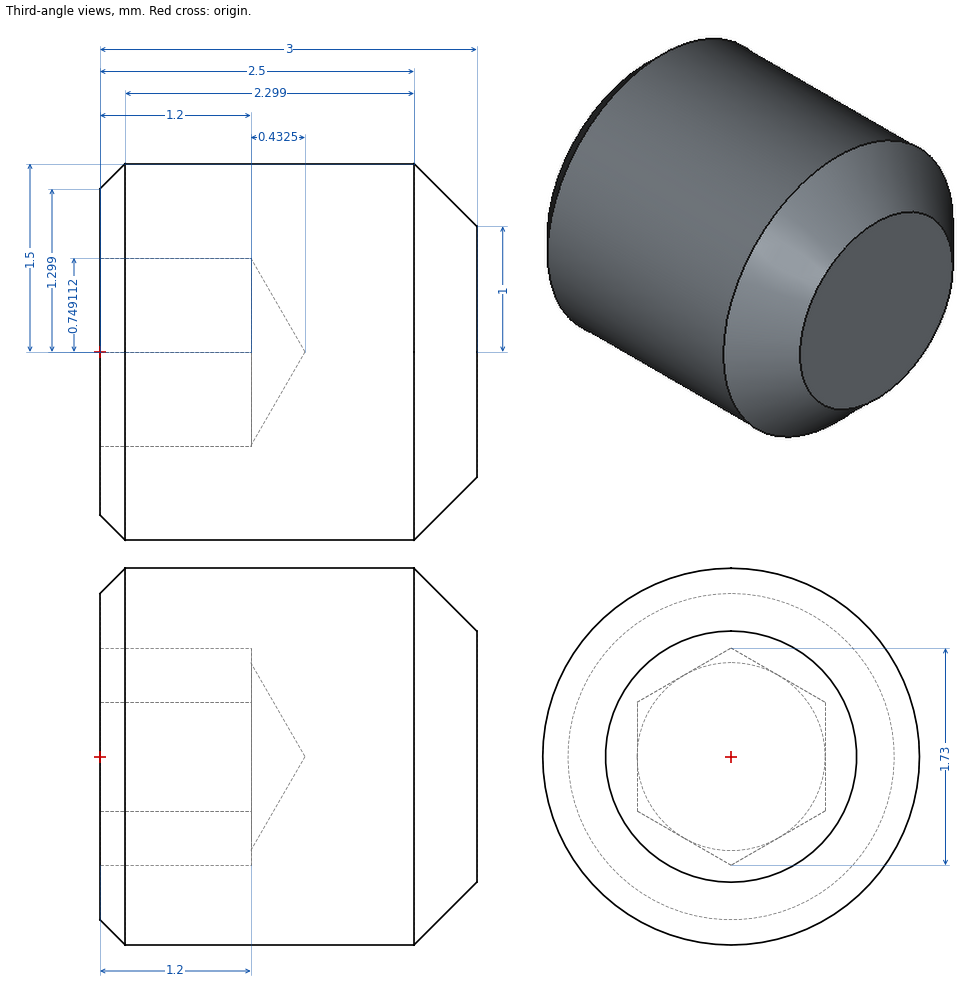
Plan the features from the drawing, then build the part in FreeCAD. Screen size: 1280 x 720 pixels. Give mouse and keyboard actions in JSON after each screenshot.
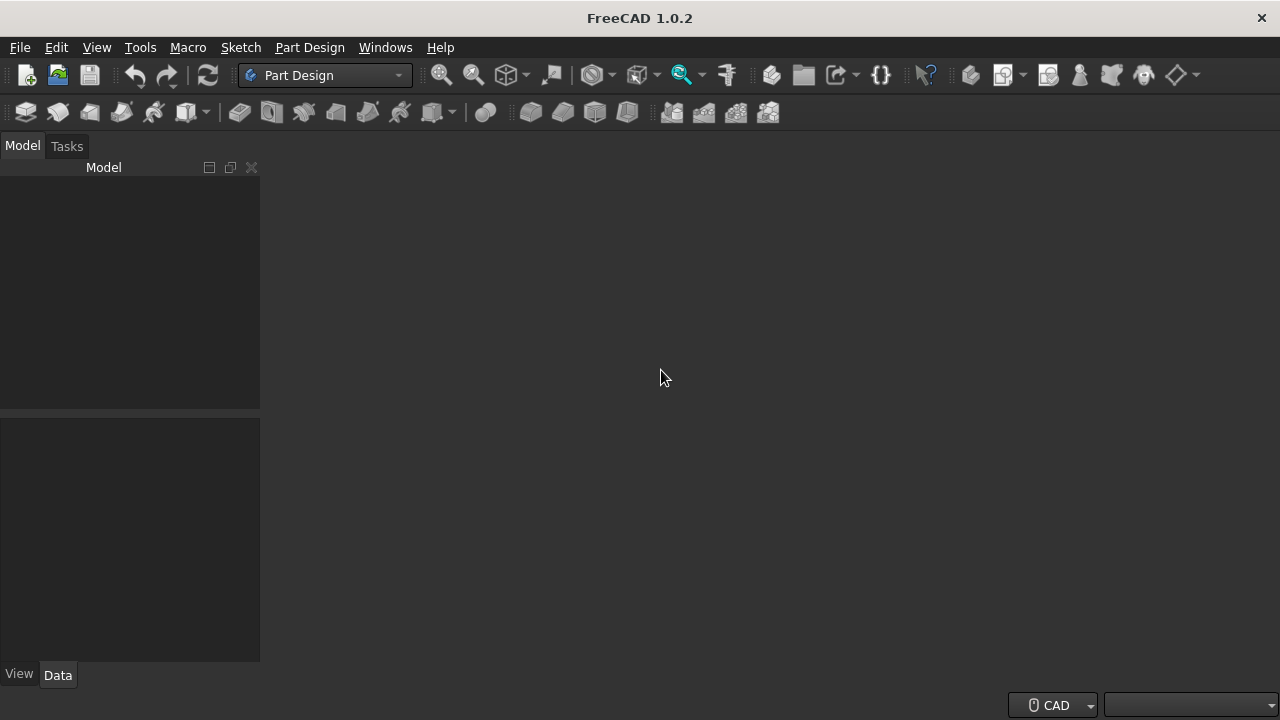
{"action": "left_click", "coordinate": [26, 76]}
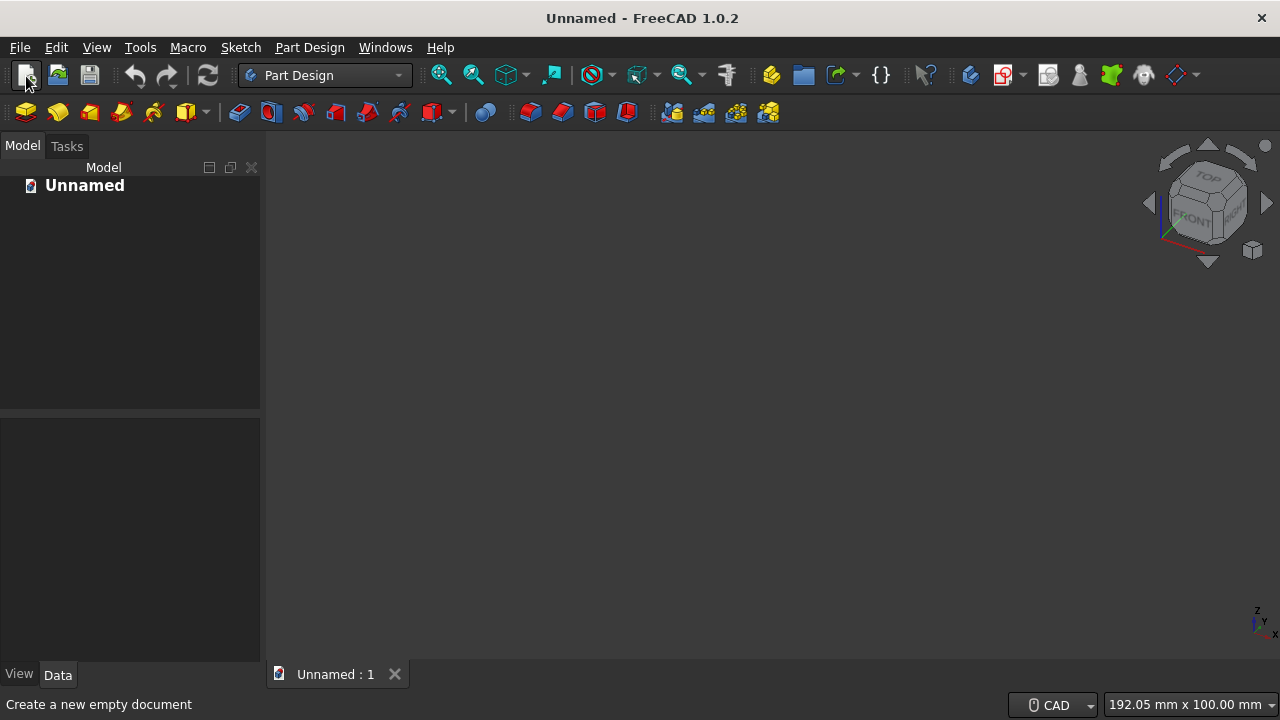
{"action": "left_click", "coordinate": [1004, 76]}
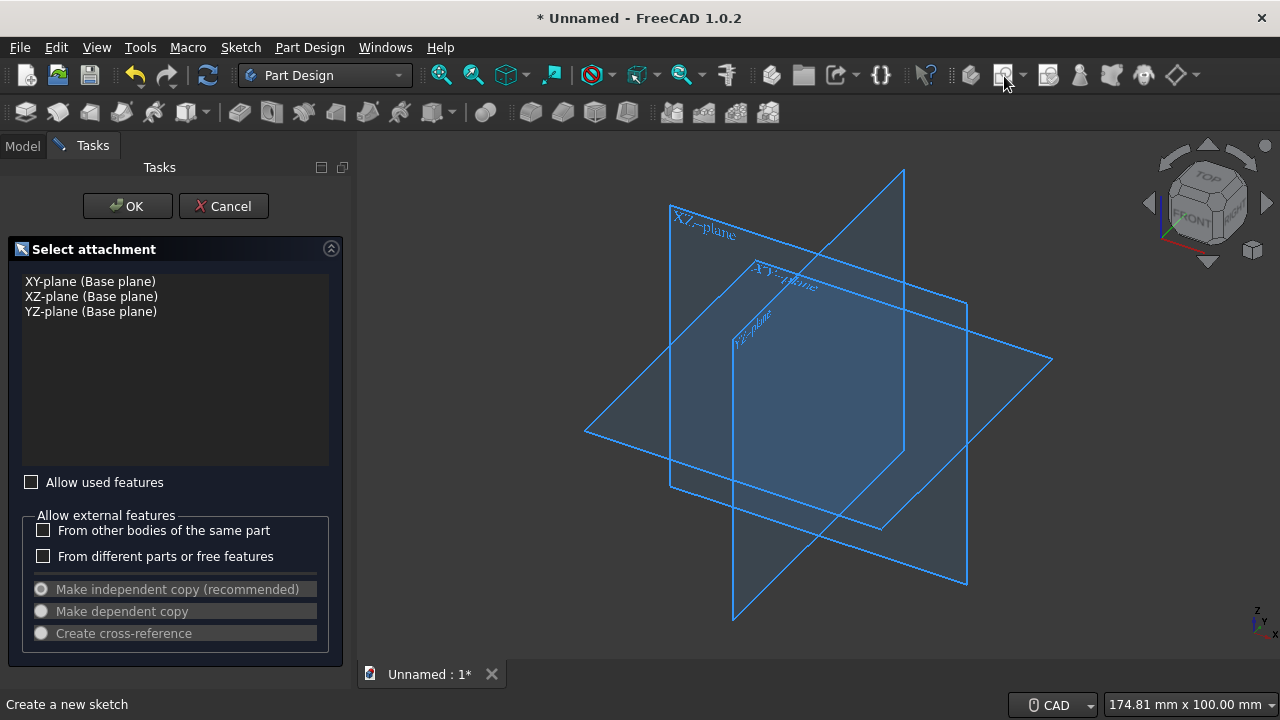
{"action": "left_click", "coordinate": [82, 282]}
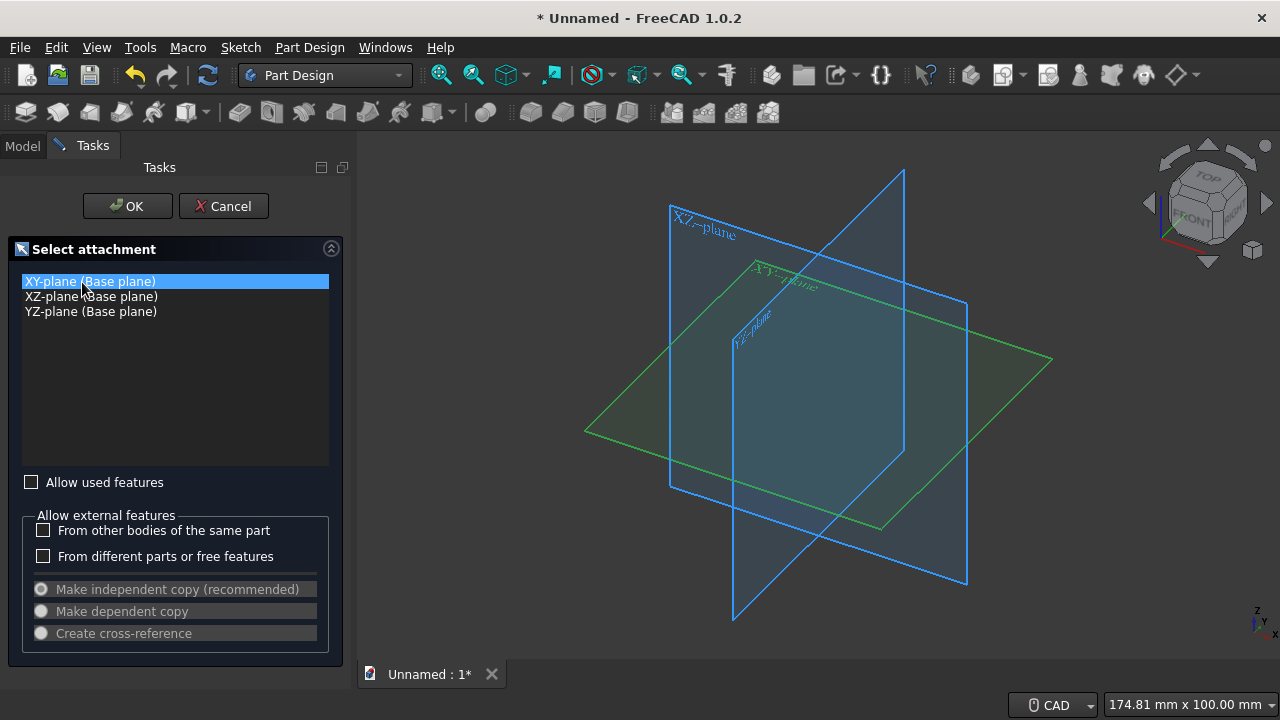
{"action": "left_click", "coordinate": [128, 206]}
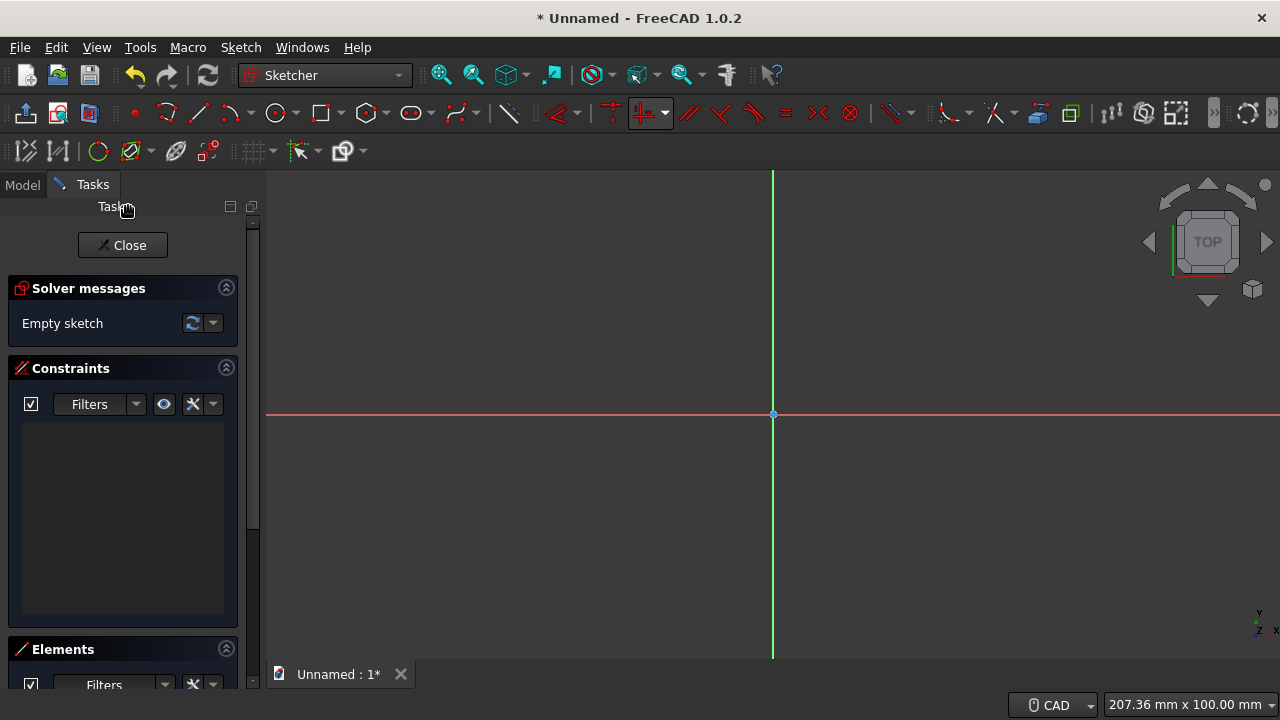
{"action": "scroll", "coordinate": [784, 411], "scroll_direction": "up", "scroll_amount": 15}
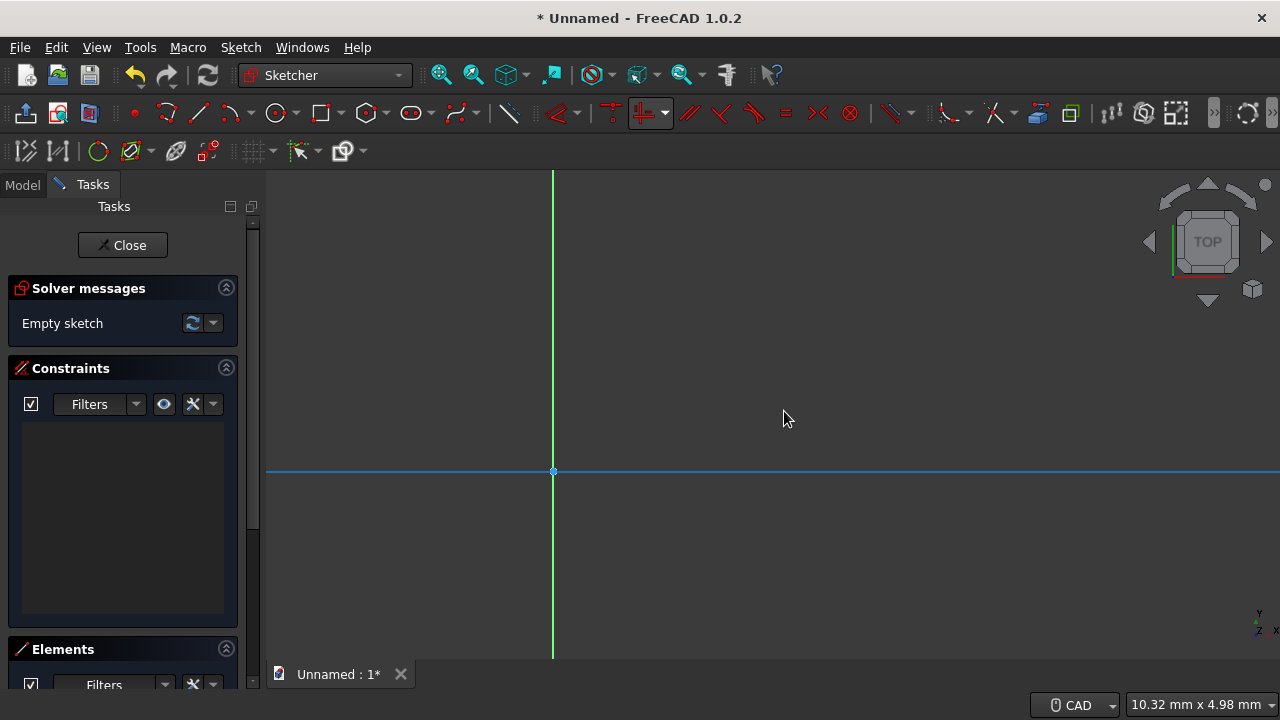
{"action": "scroll", "coordinate": [696, 378], "scroll_direction": "up", "scroll_amount": 3}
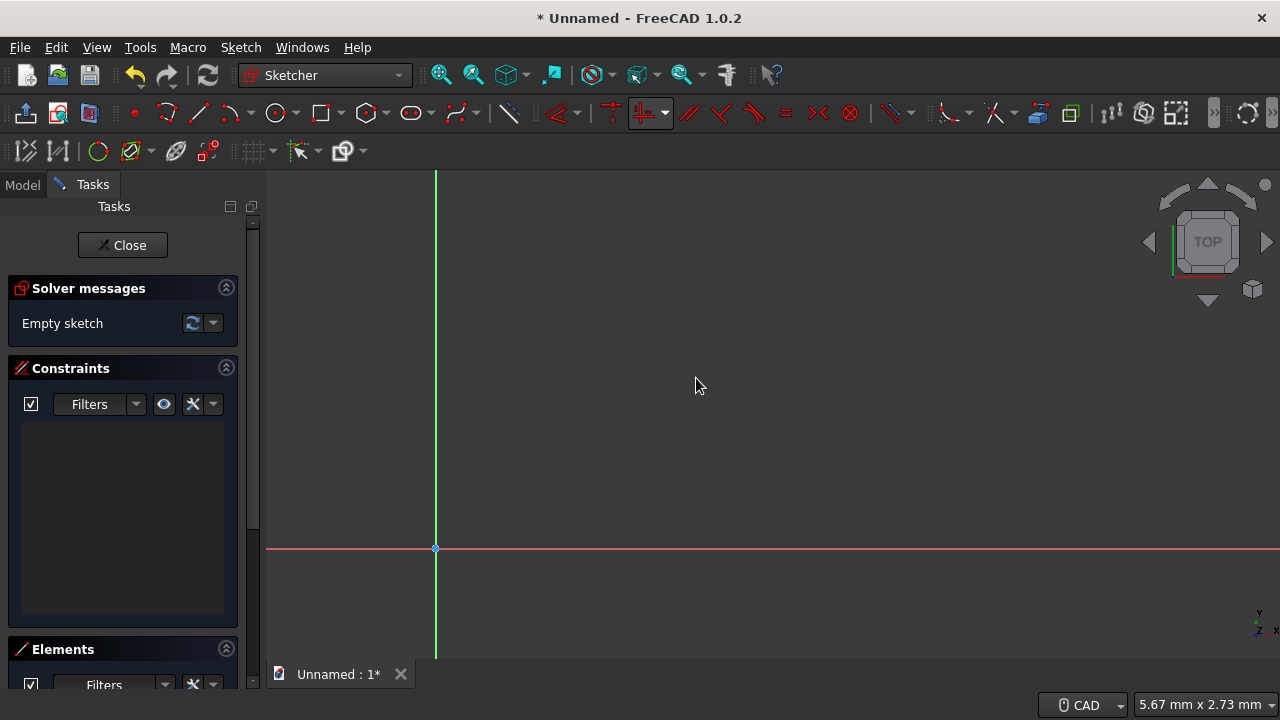
{"action": "left_click", "coordinate": [168, 114]}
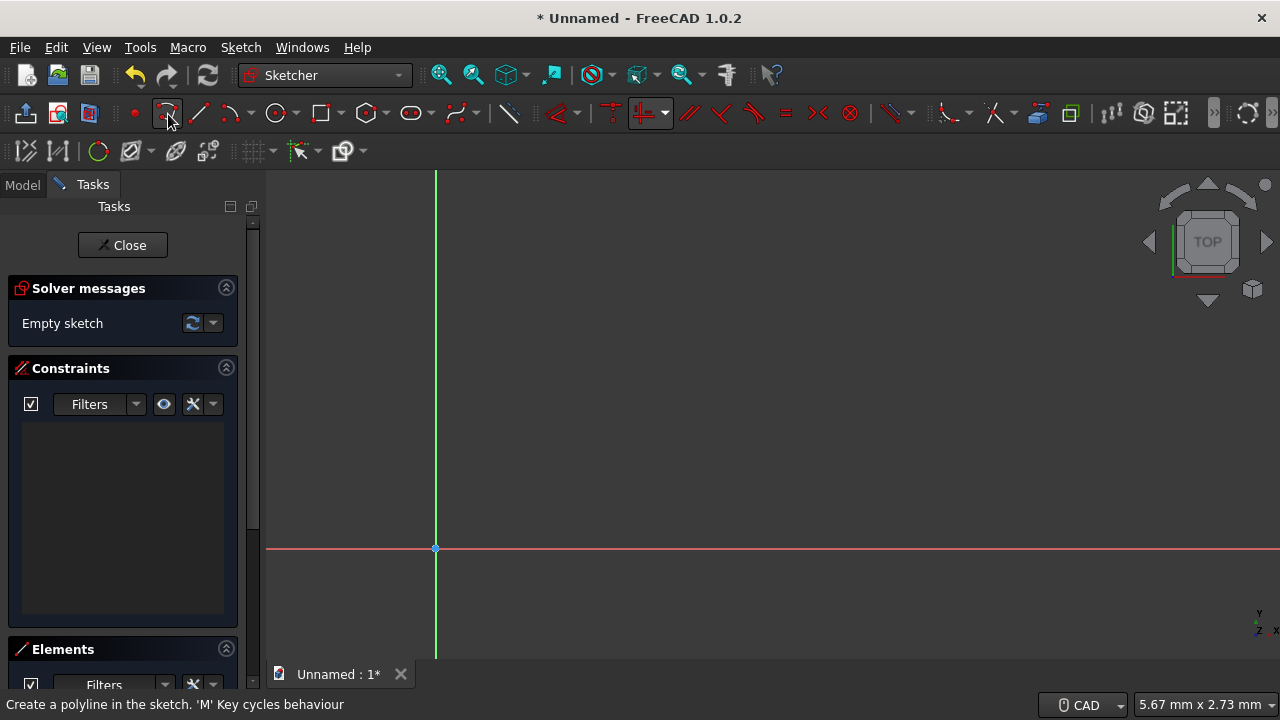
{"action": "left_click", "coordinate": [436, 549]}
{"action": "left_click", "coordinate": [973, 540]}
{"action": "left_click", "coordinate": [973, 370]}
{"action": "left_click", "coordinate": [883, 280]}
{"action": "left_click", "coordinate": [472, 280]}
{"action": "left_click", "coordinate": [445, 316]}
{"action": "left_click", "coordinate": [436, 549]}
{"action": "key", "text": "Escape"}
{"action": "key", "text": "Escape"}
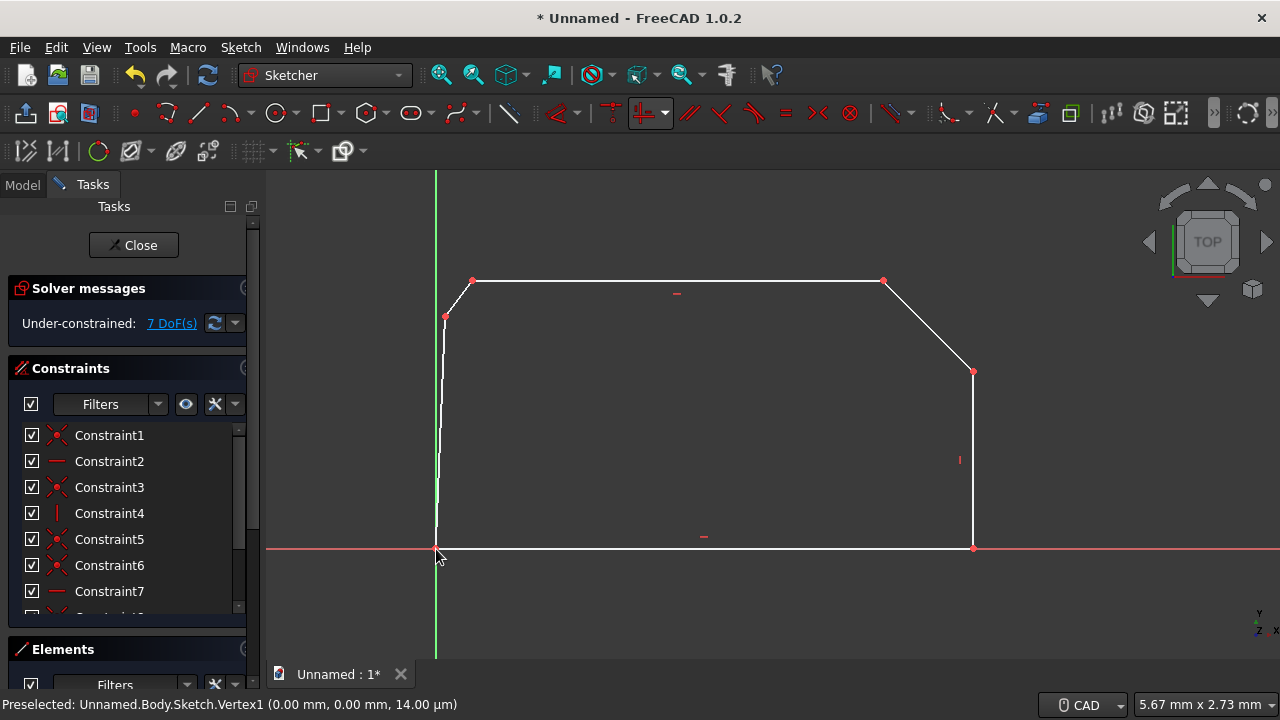
{"action": "left_click", "coordinate": [438, 479]}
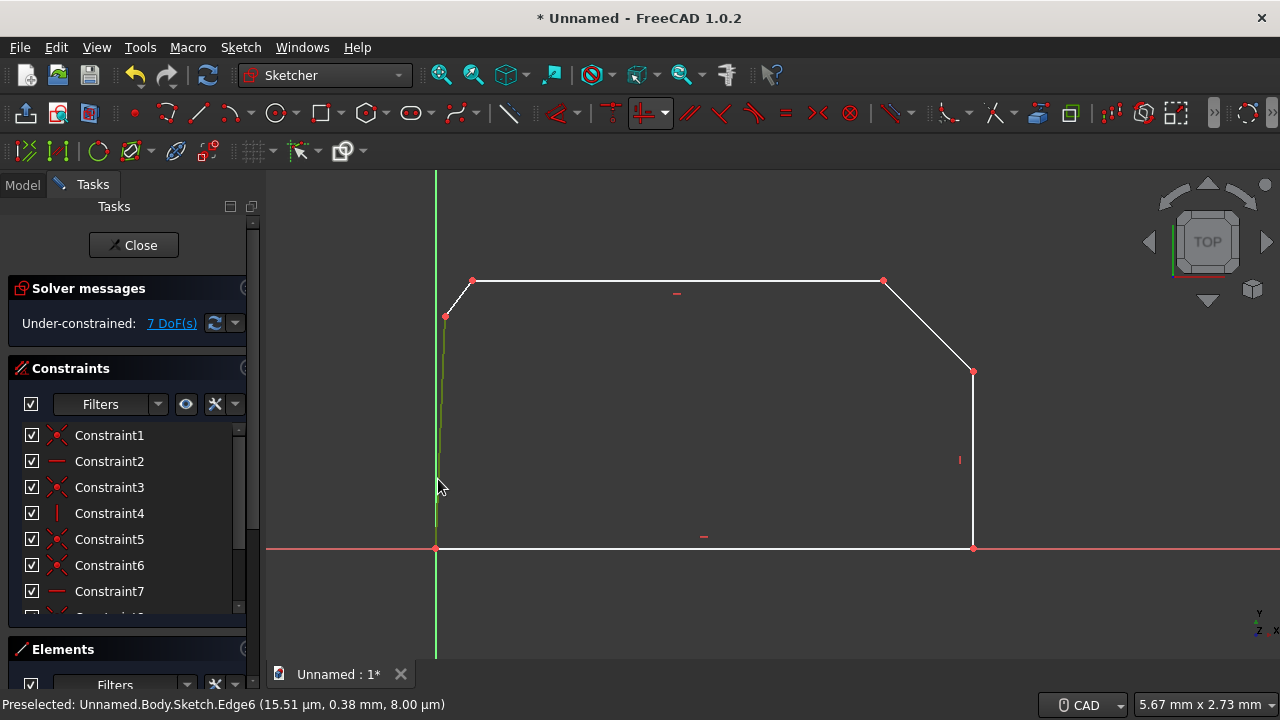
{"action": "key", "text": "v"}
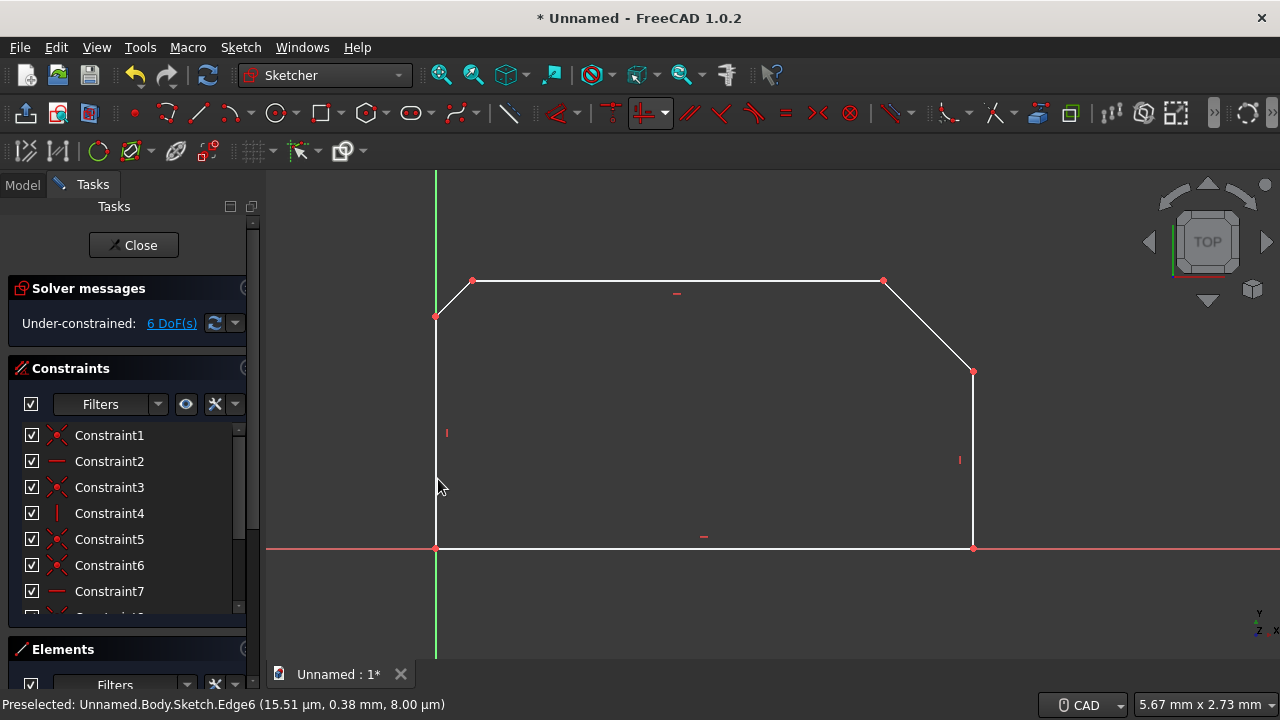
{"action": "left_click", "coordinate": [597, 549]}